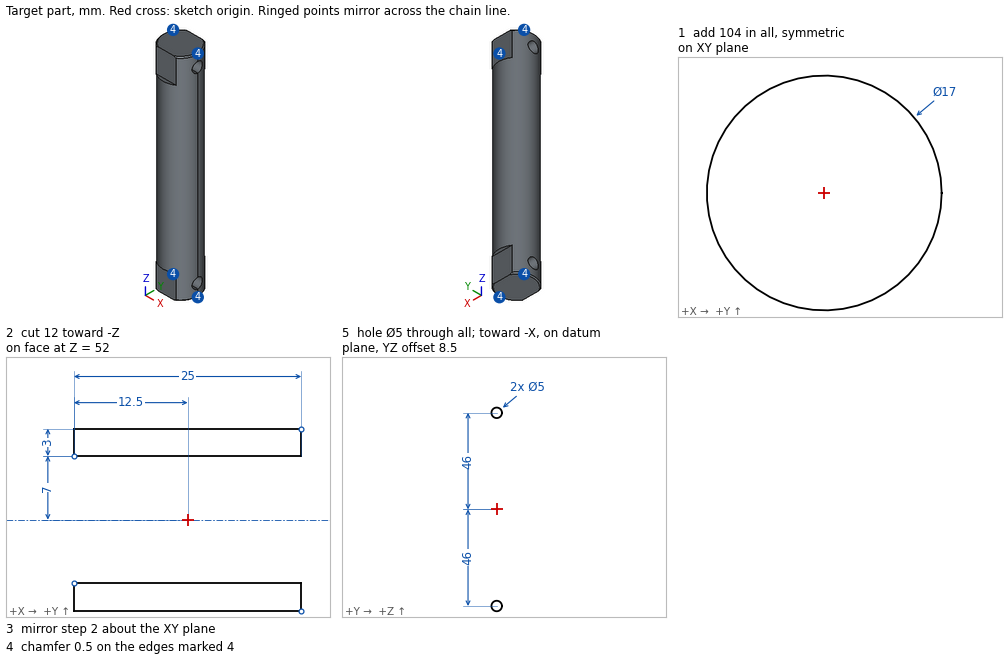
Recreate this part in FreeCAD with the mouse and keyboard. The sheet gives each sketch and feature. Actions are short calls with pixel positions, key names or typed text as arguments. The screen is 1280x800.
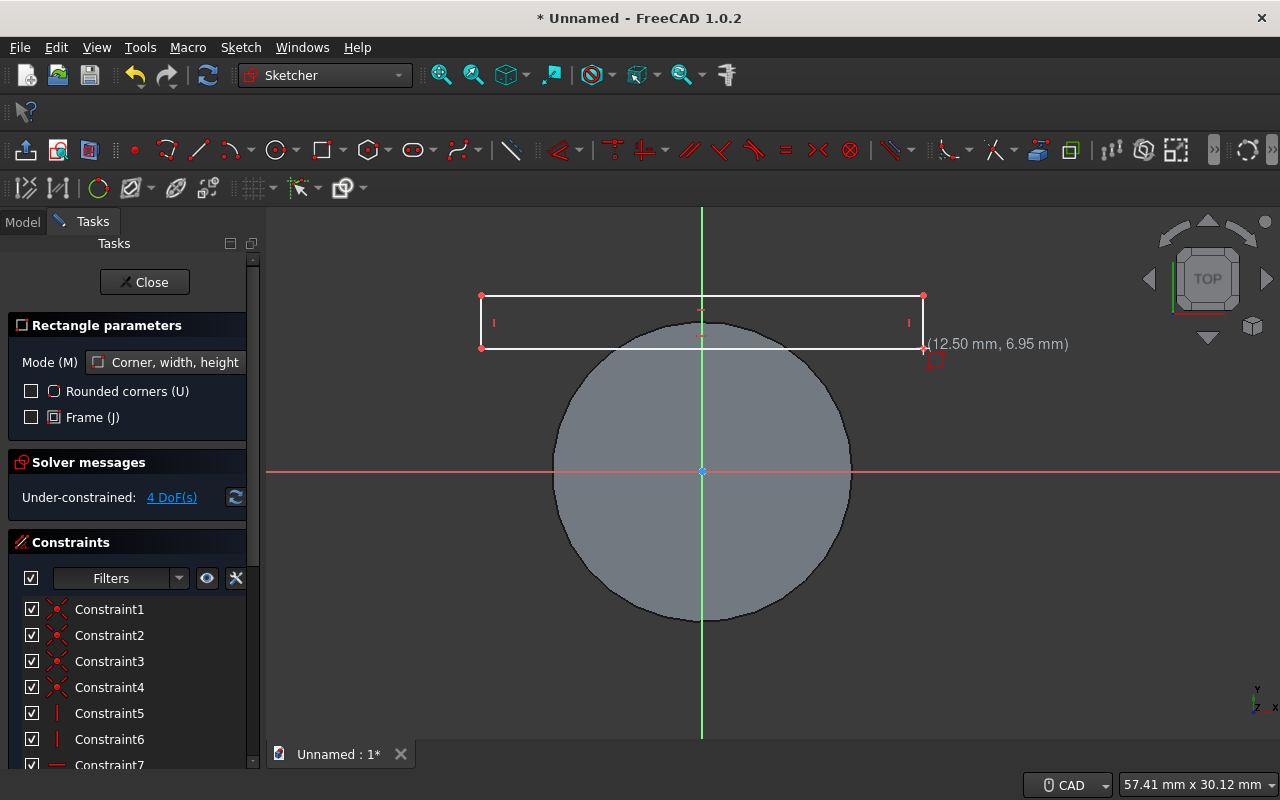
click(481, 595)
click(923, 648)
key(Escape)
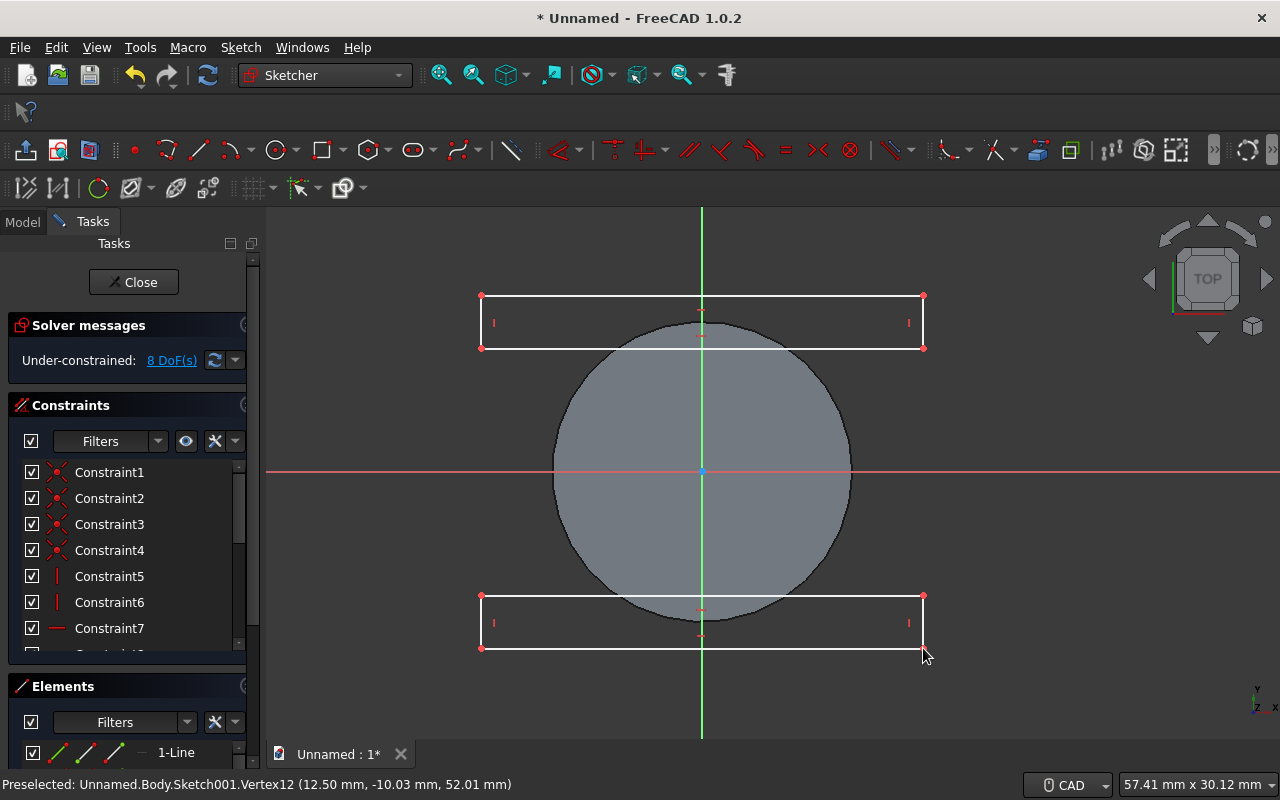
click(481, 349)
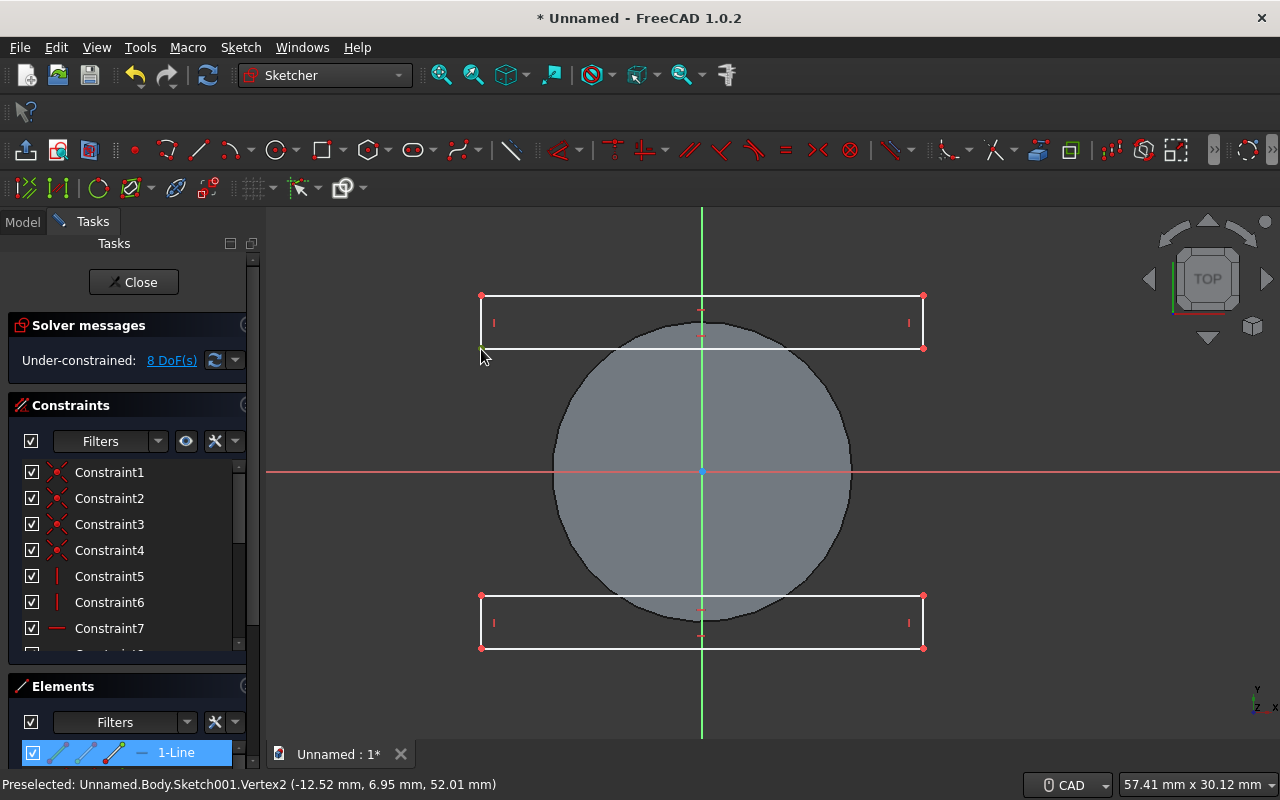
click(481, 596)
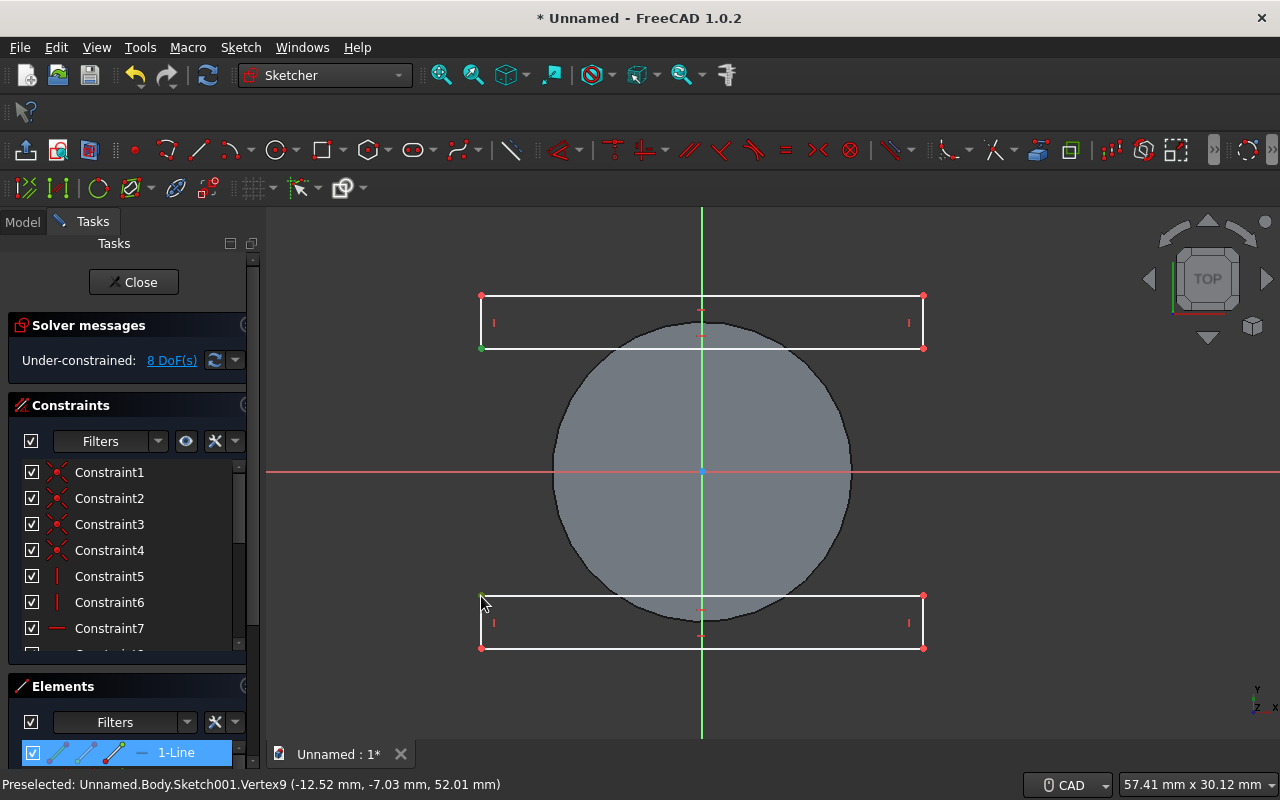
click(353, 472)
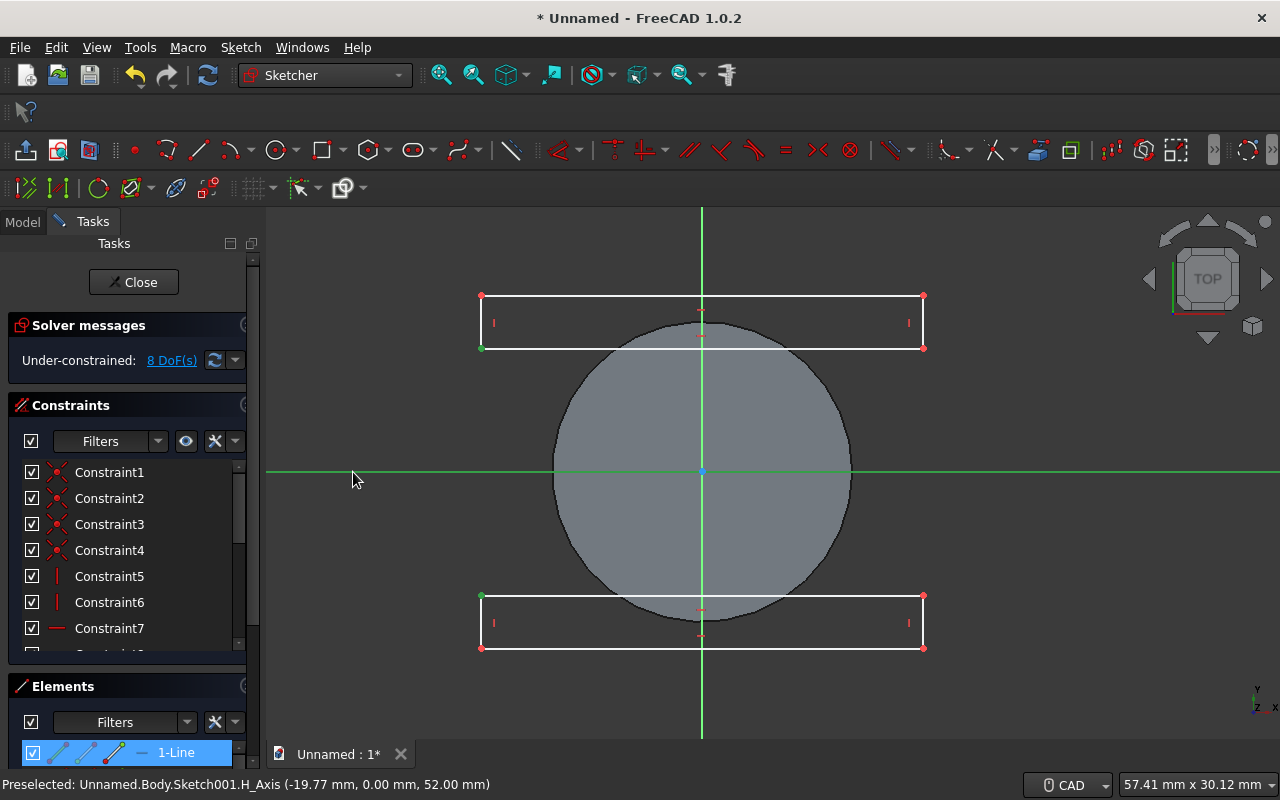
click(818, 150)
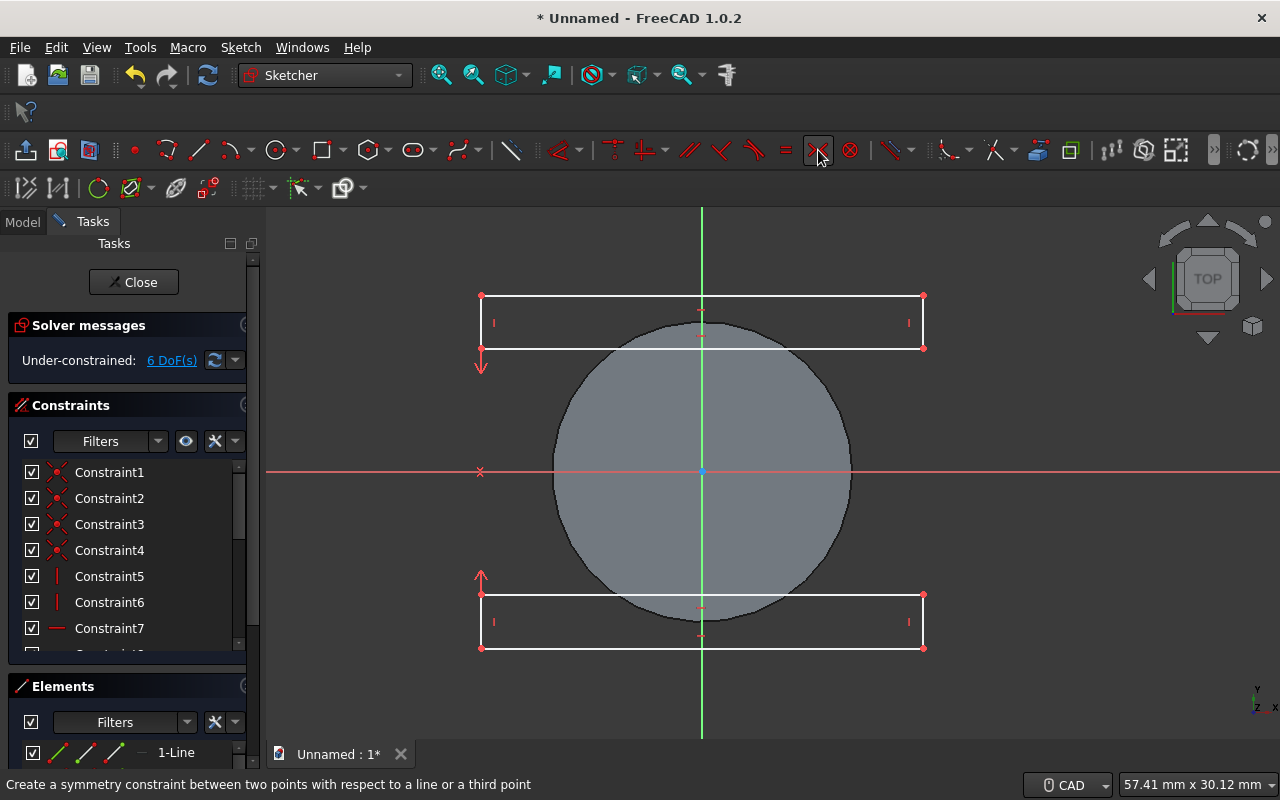
click(923, 296)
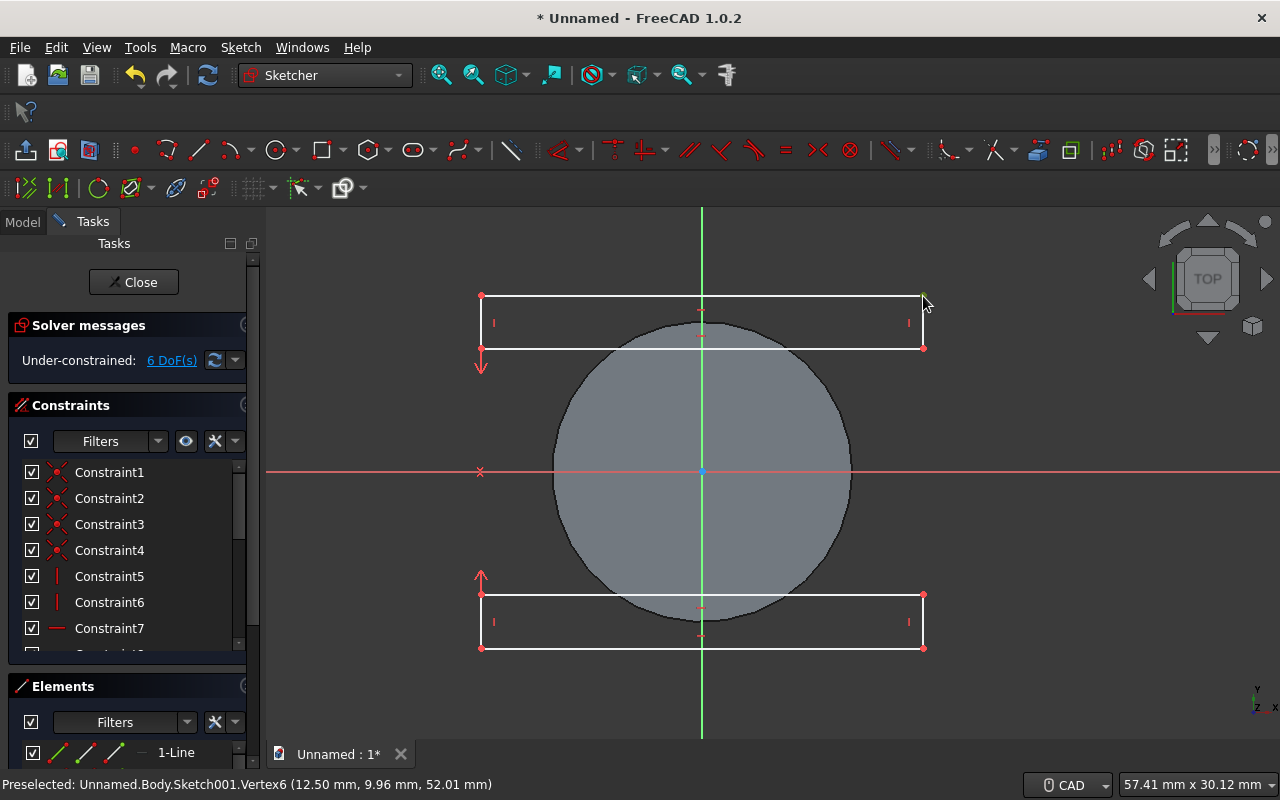
click(923, 649)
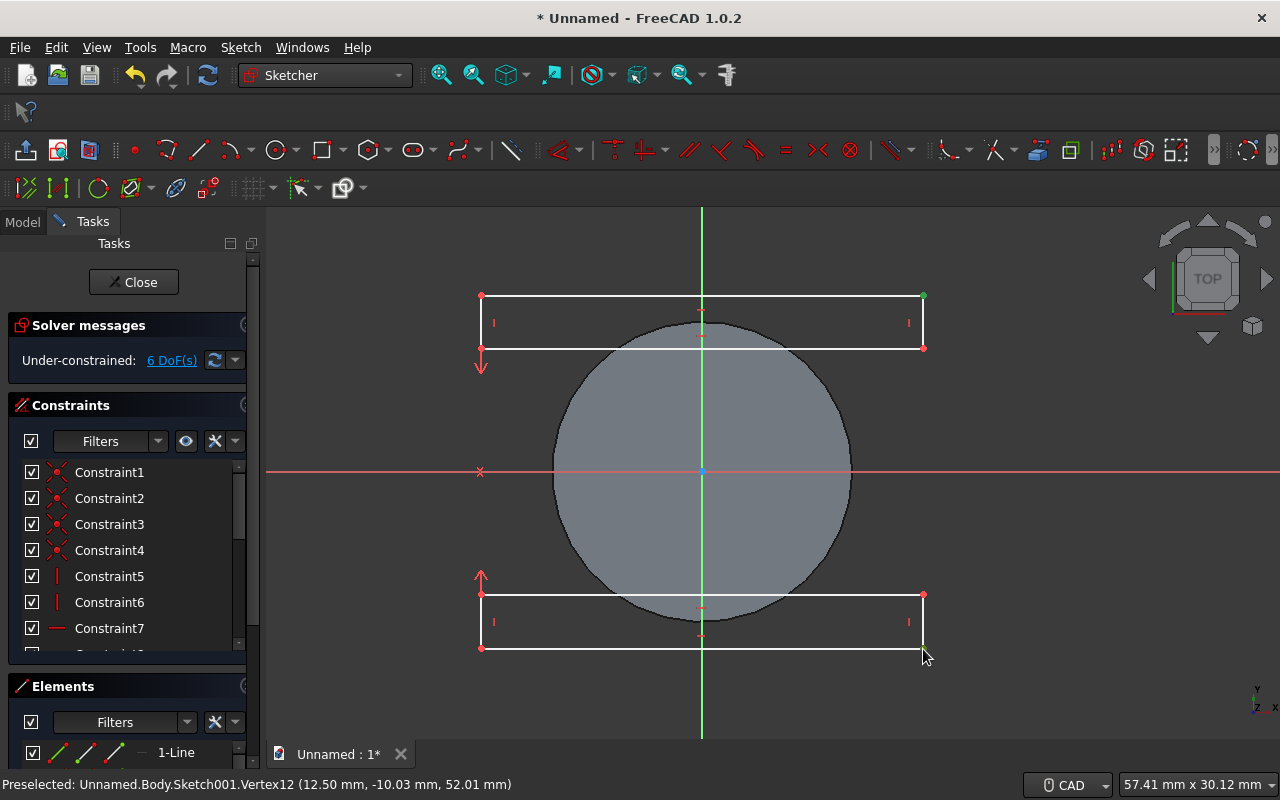
click(353, 472)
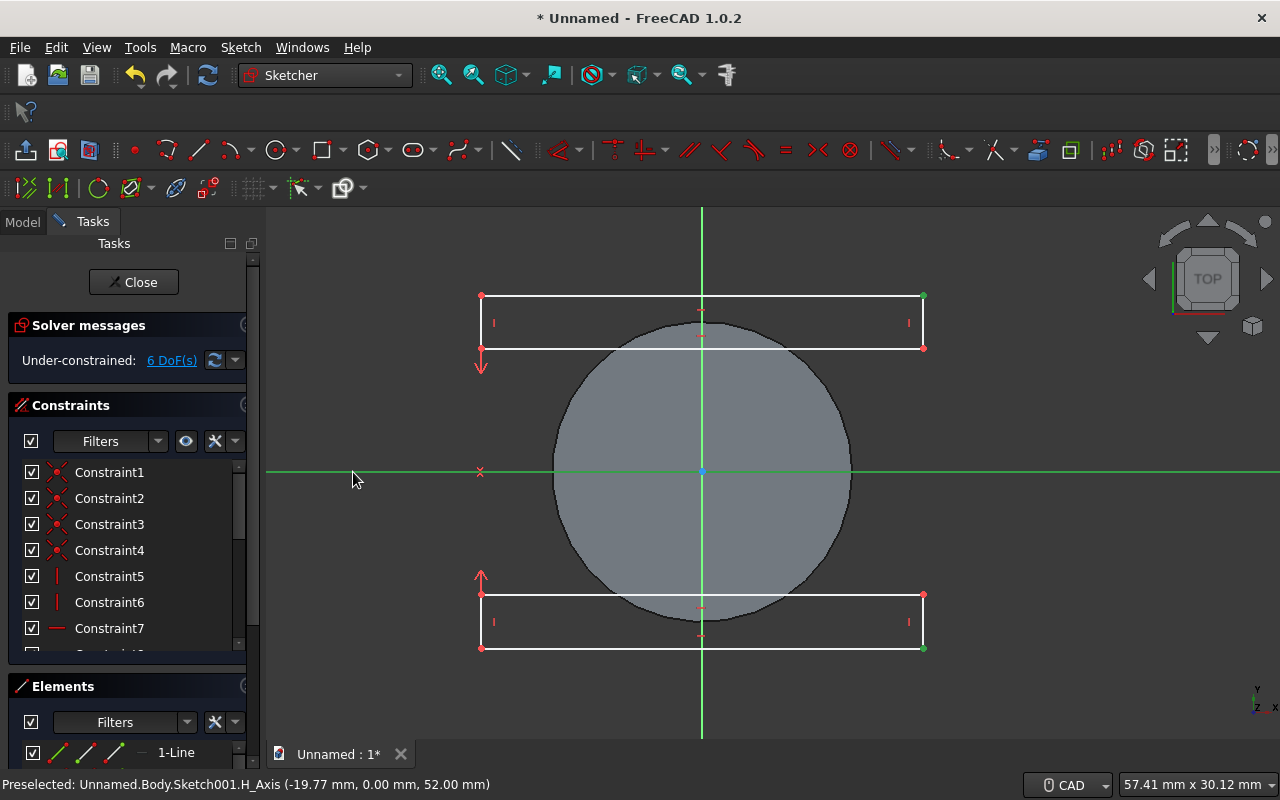
click(818, 150)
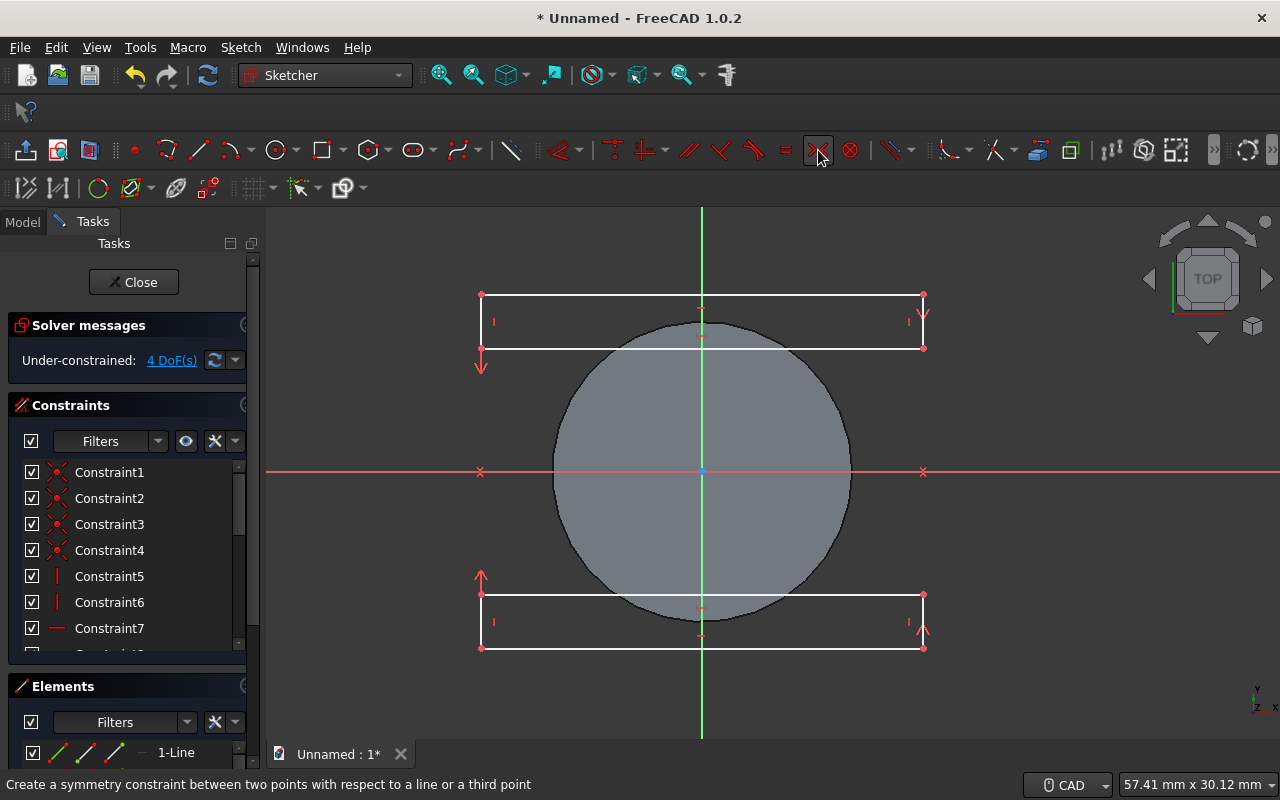
click(558, 150)